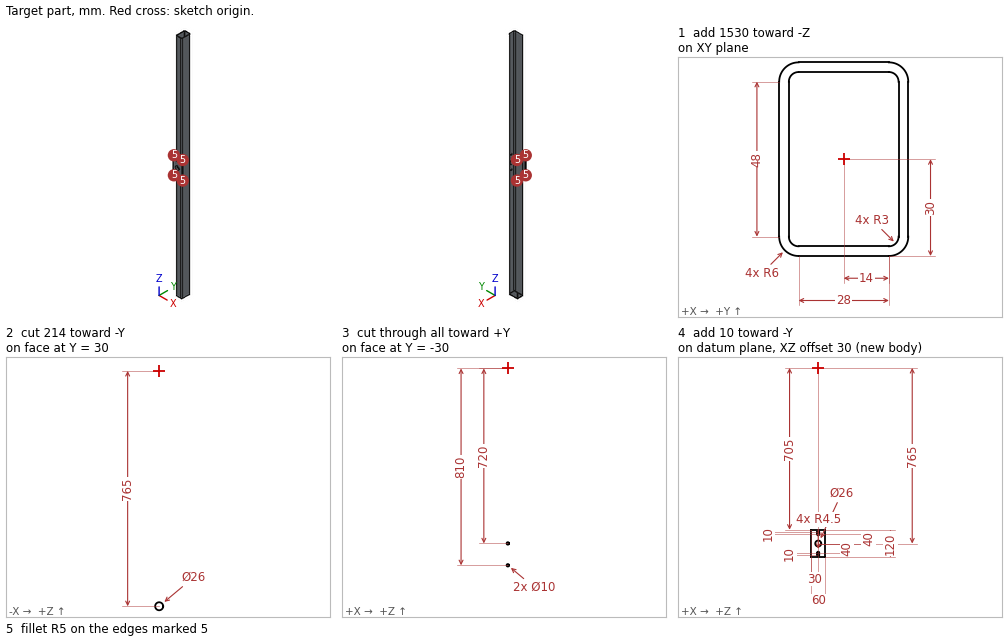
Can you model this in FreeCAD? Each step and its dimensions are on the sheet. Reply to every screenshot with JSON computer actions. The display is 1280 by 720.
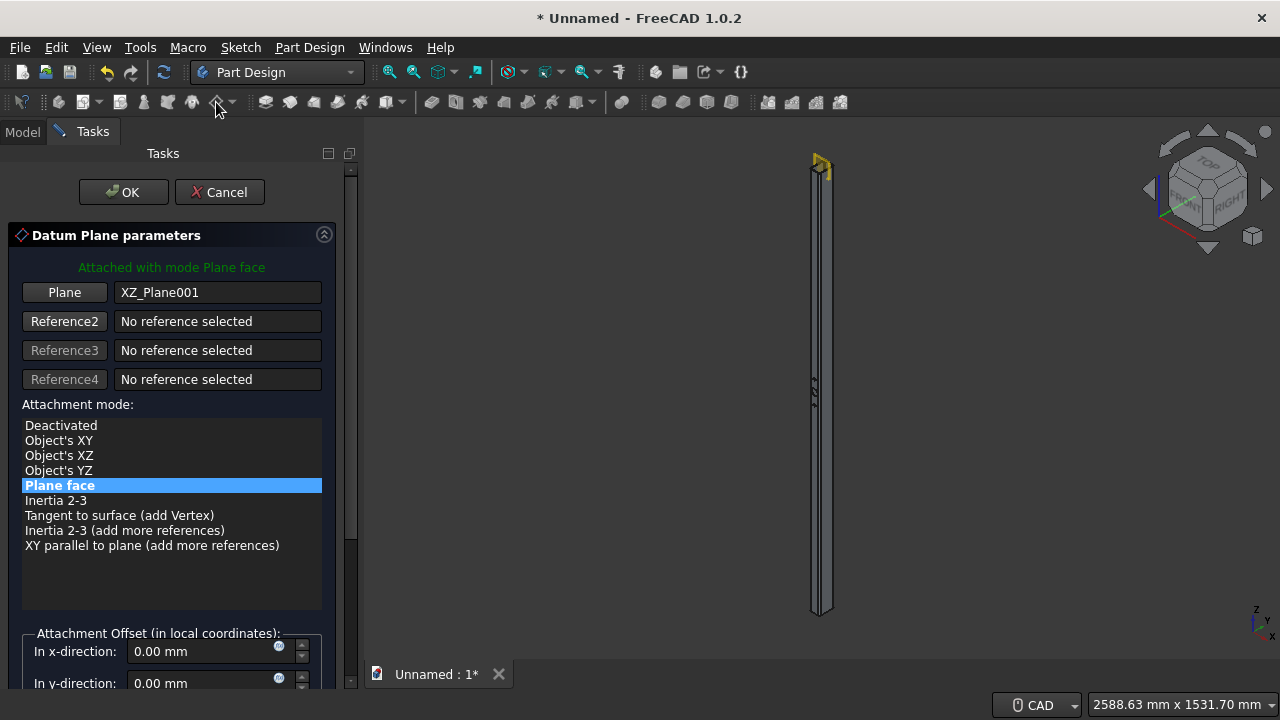
{"action": "scroll", "coordinate": [351, 426], "scroll_direction": "down", "scroll_amount": 2}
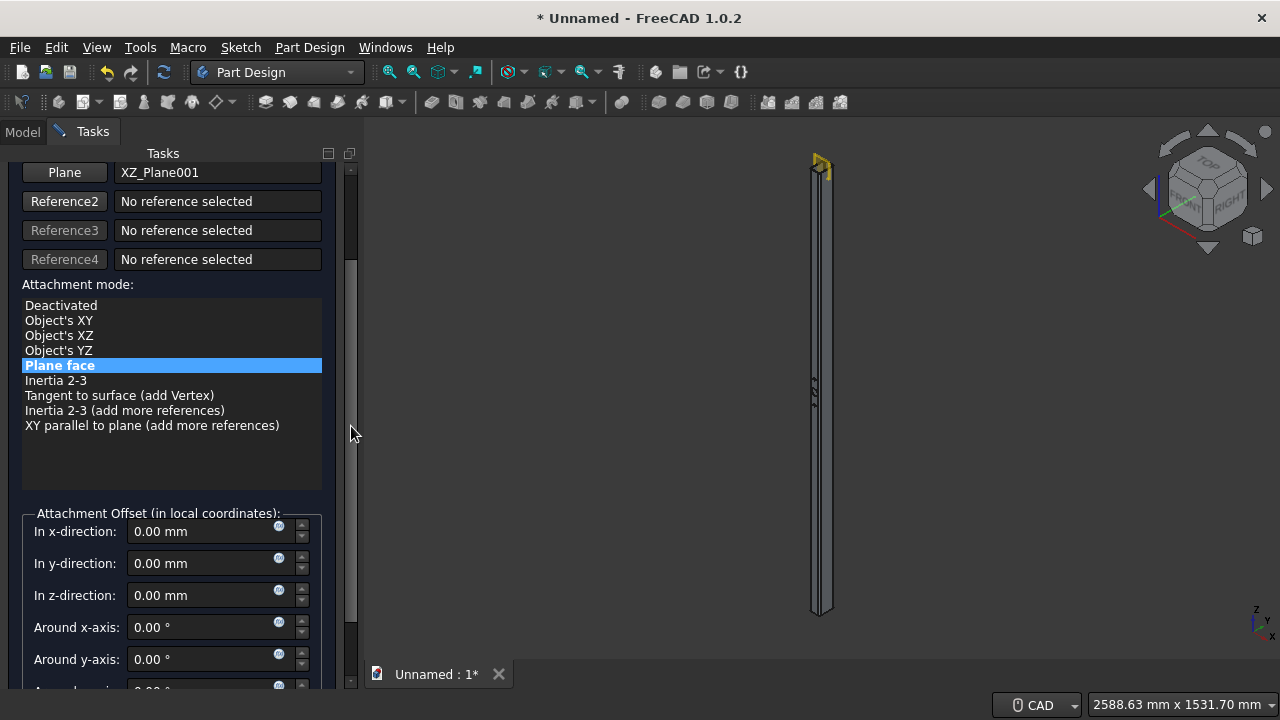
{"action": "triple_click", "coordinate": [210, 595]}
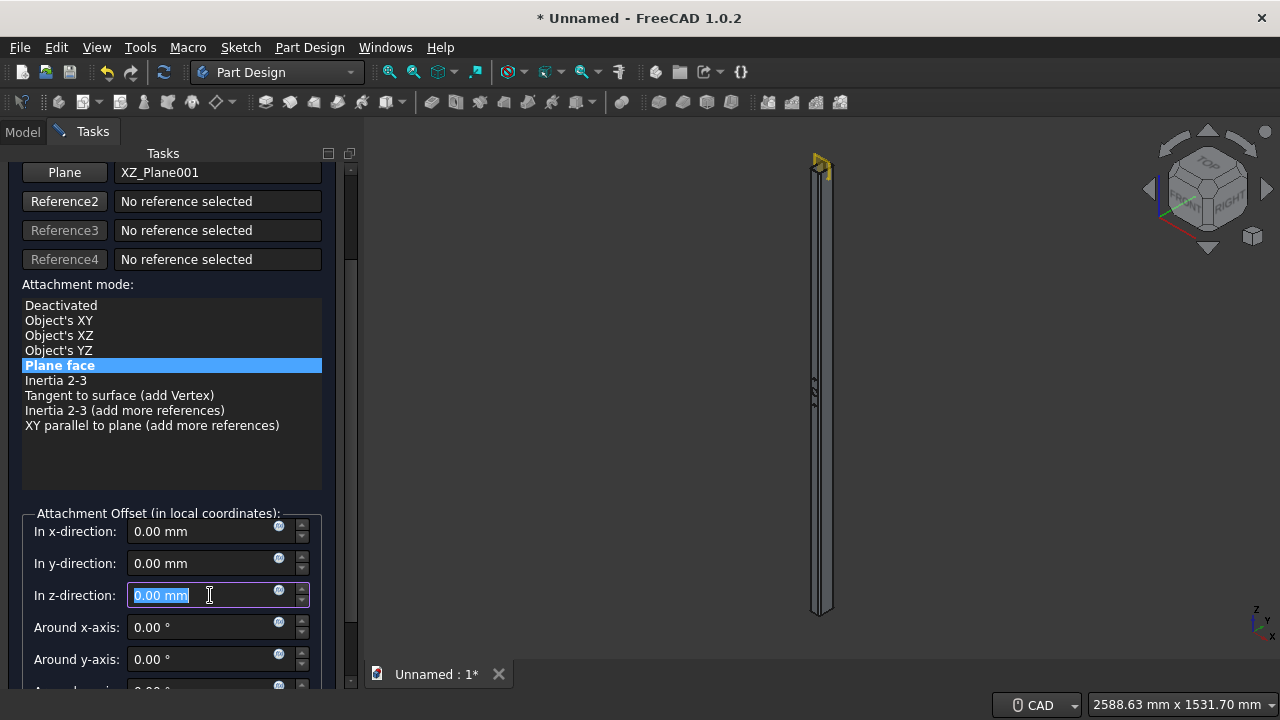
{"action": "type", "text": "30"}
{"action": "key", "text": "Tab"}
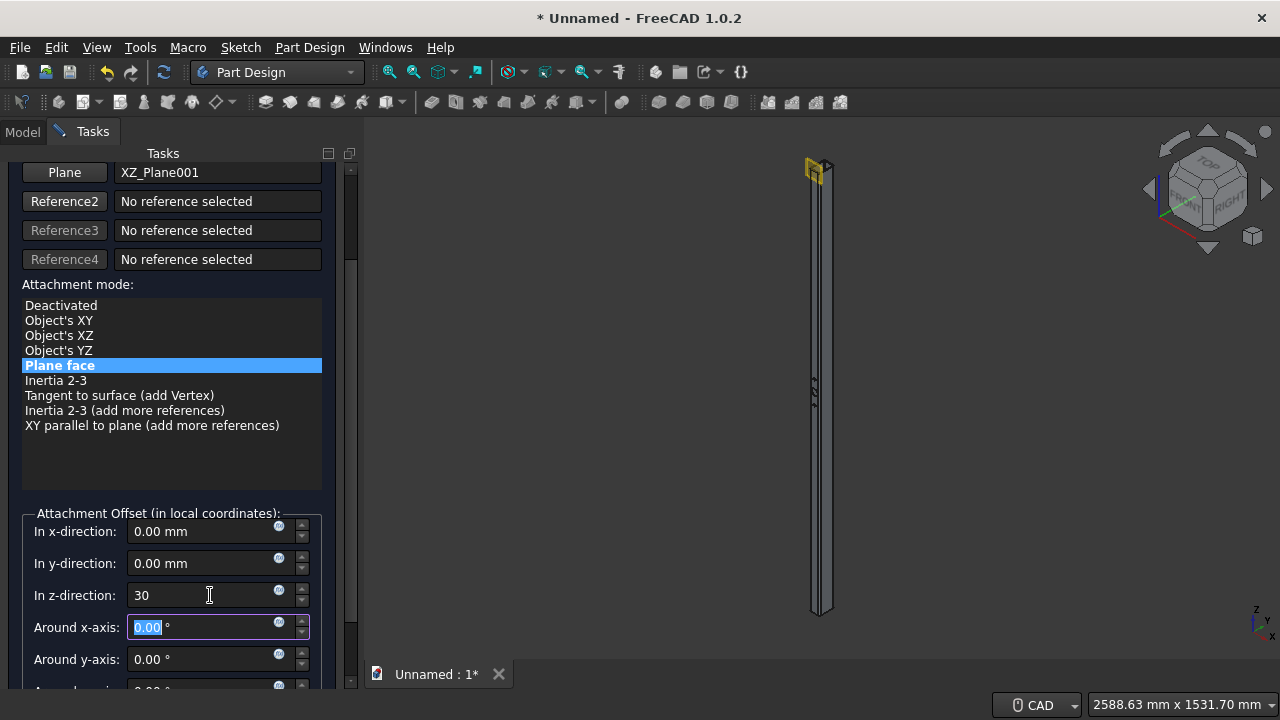
{"action": "scroll", "coordinate": [351, 426], "scroll_direction": "up", "scroll_amount": 3}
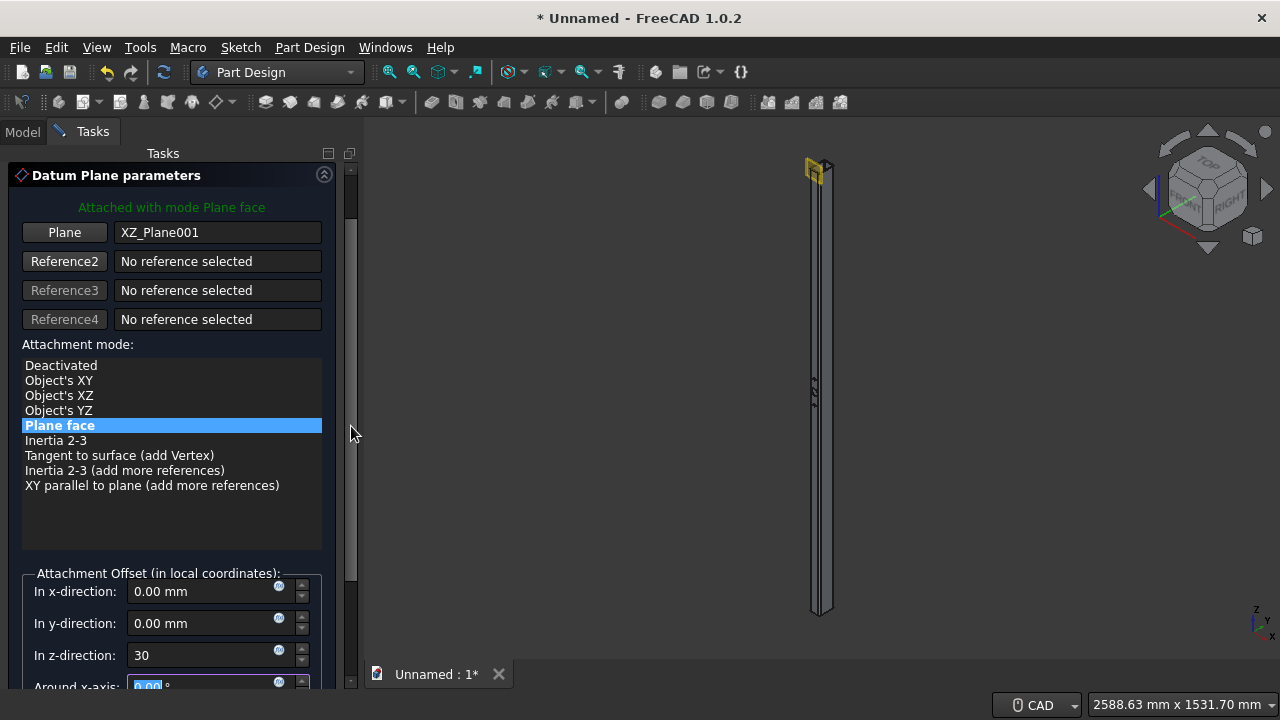
{"action": "left_click", "coordinate": [124, 192]}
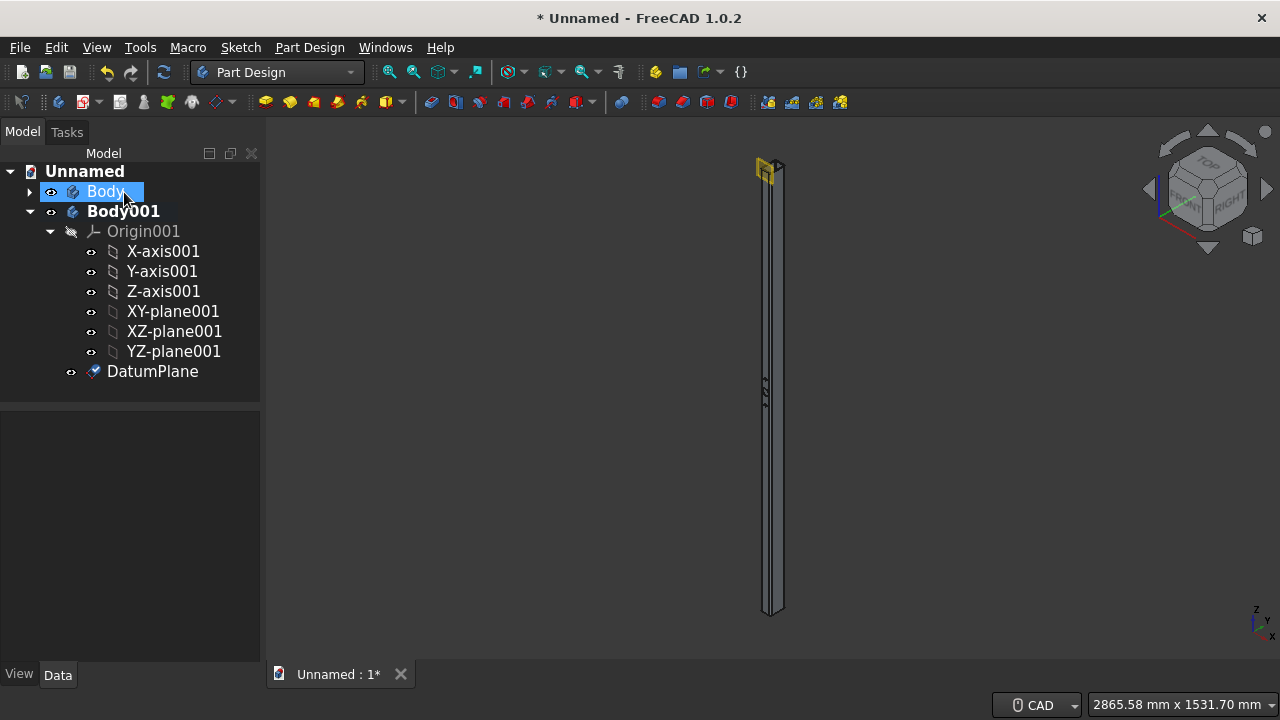
{"action": "left_click", "coordinate": [116, 372]}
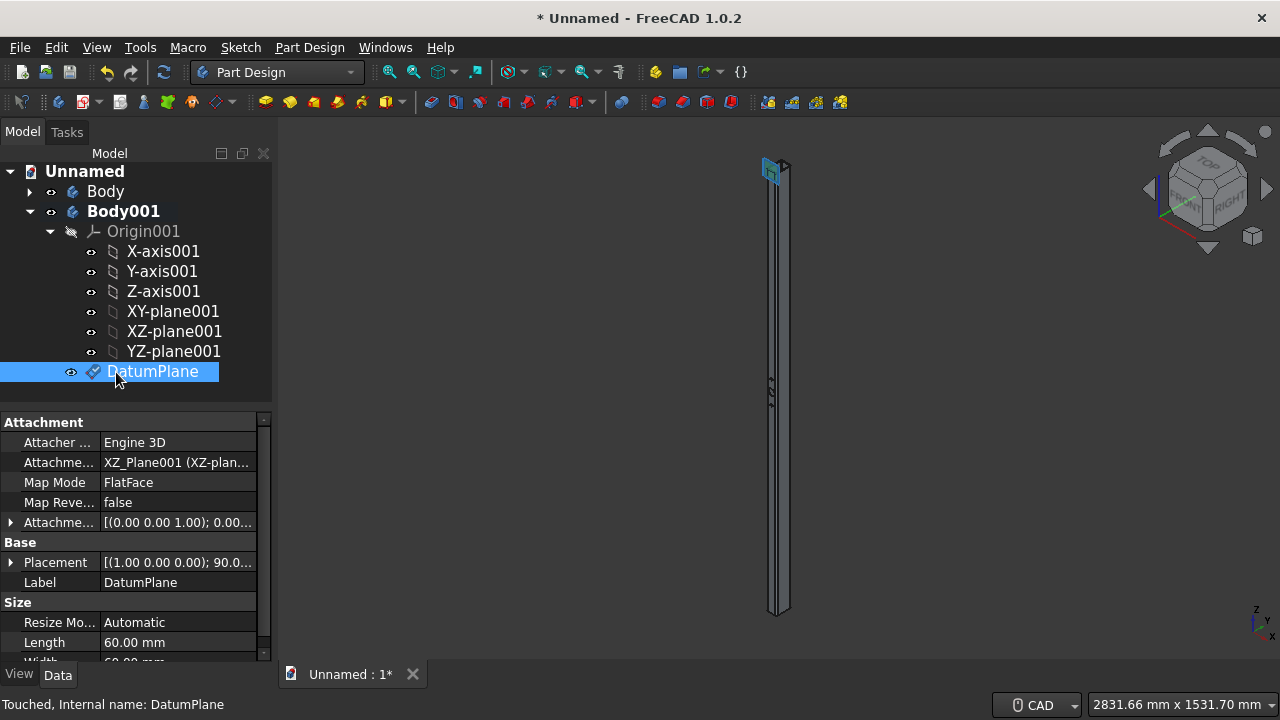
{"action": "left_click", "coordinate": [84, 102]}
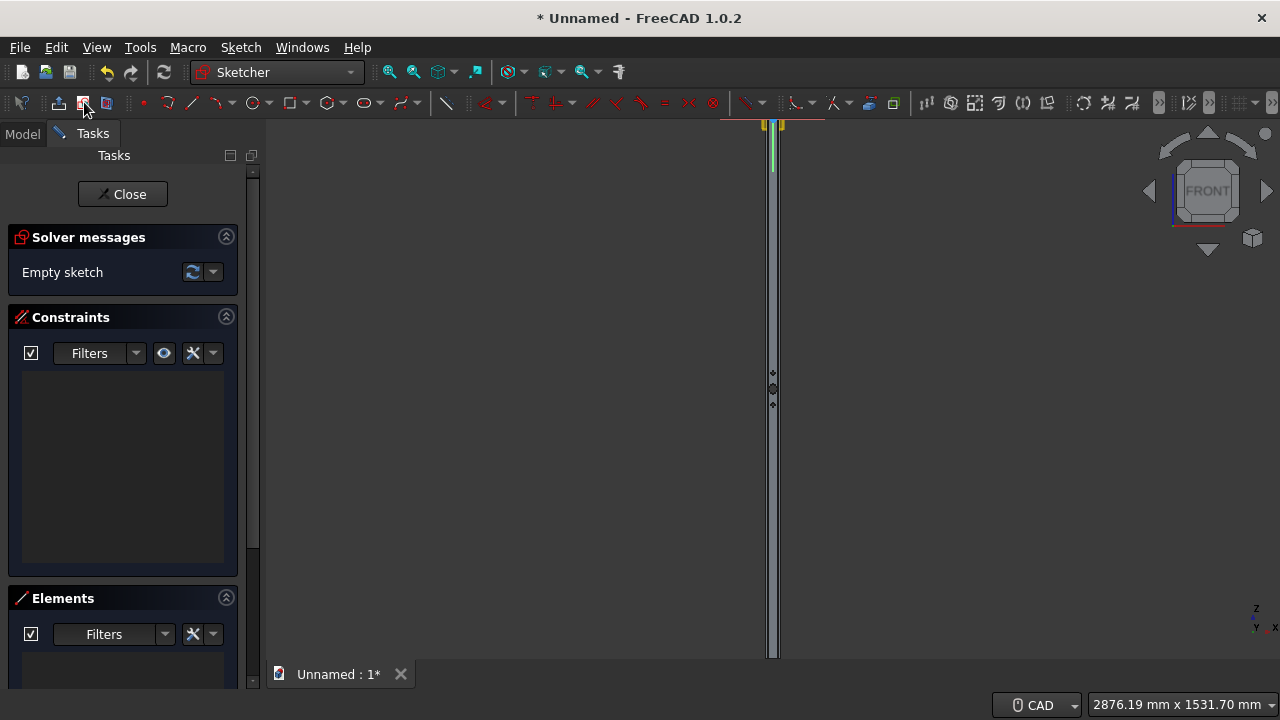
{"action": "scroll", "coordinate": [784, 389], "scroll_direction": "up", "scroll_amount": 10}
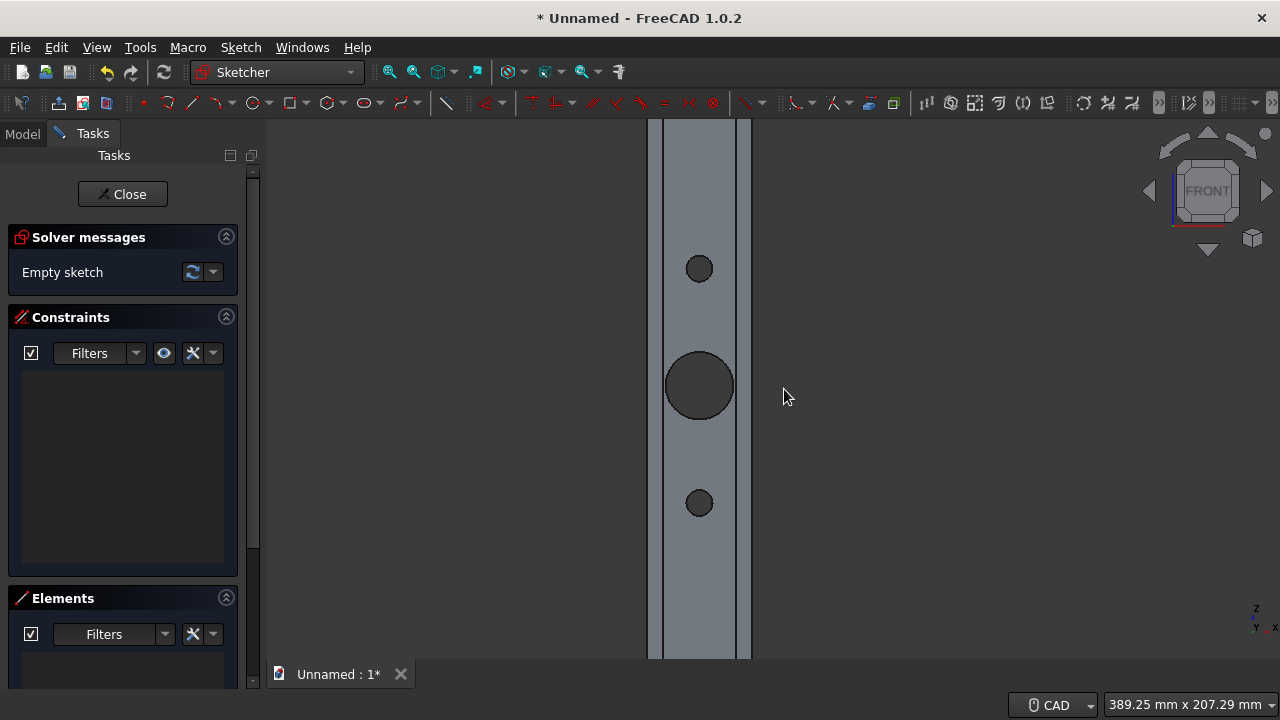
{"action": "left_click", "coordinate": [290, 104]}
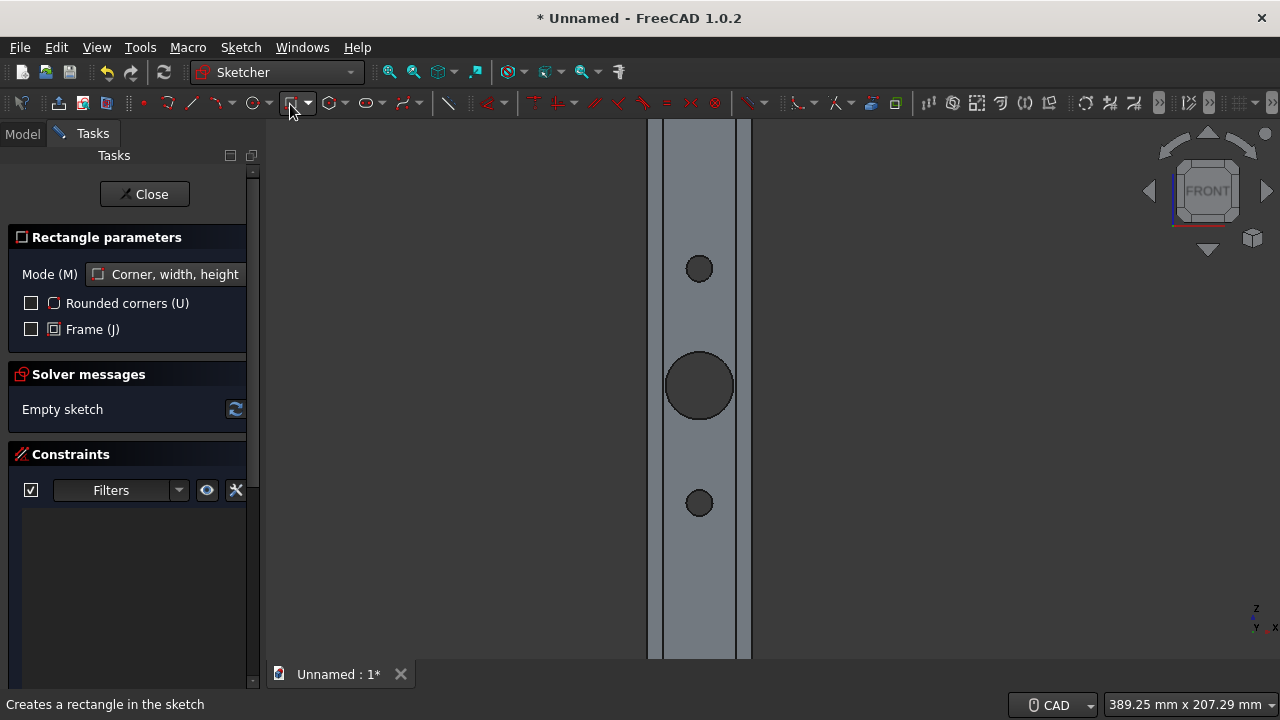
{"action": "left_click", "coordinate": [621, 229]}
{"action": "mouse_move", "coordinate": [778, 542]}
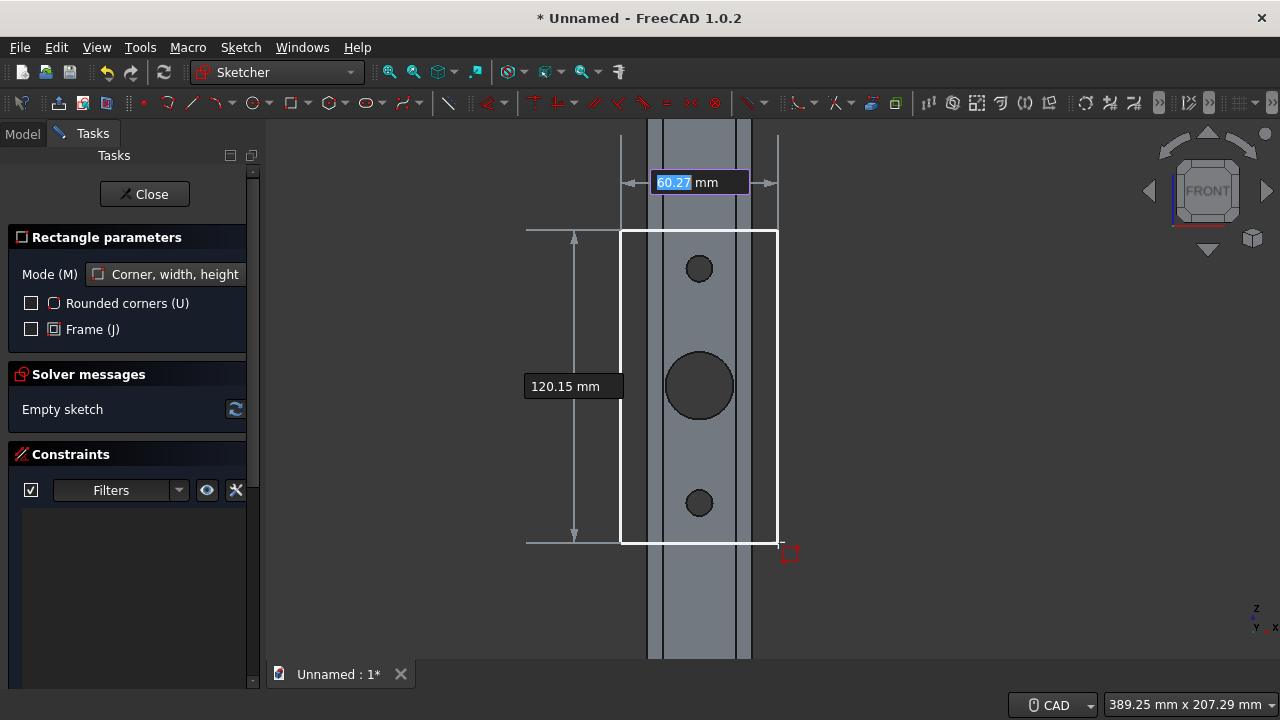
{"action": "type", "text": "60"}
{"action": "key", "text": "Tab"}
{"action": "type", "text": "120"}
{"action": "key", "text": "Return"}